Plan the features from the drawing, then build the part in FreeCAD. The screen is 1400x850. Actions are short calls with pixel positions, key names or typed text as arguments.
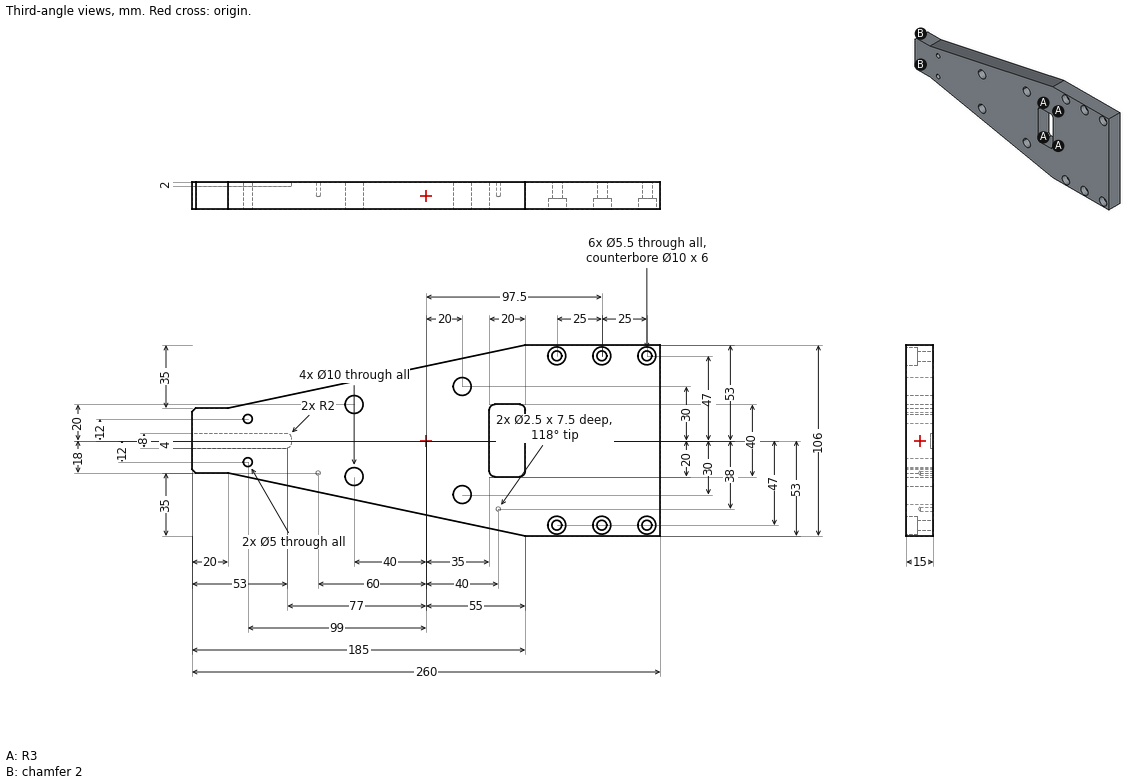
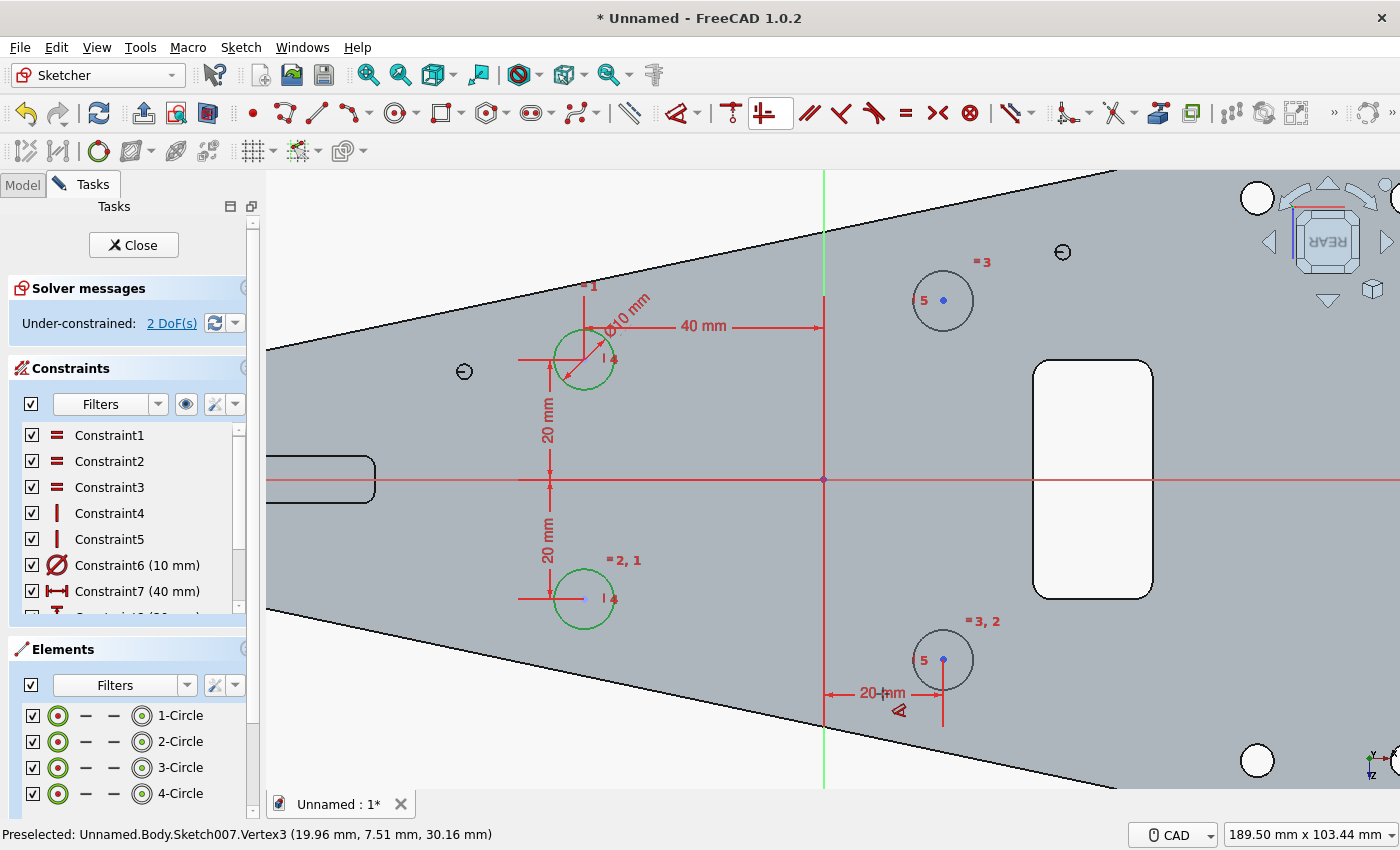
click(943, 660)
click(977, 570)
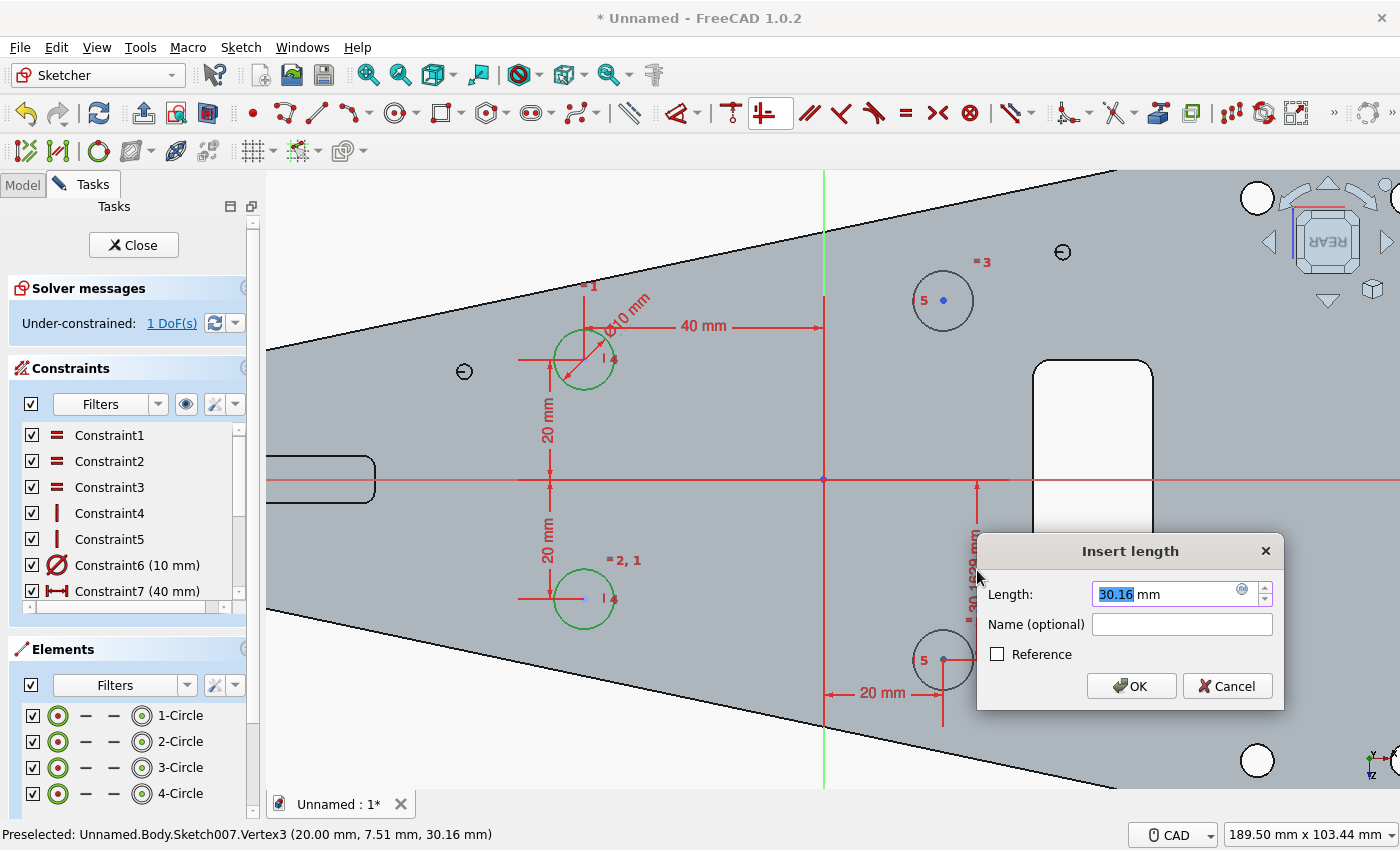
text(30)
key(Return)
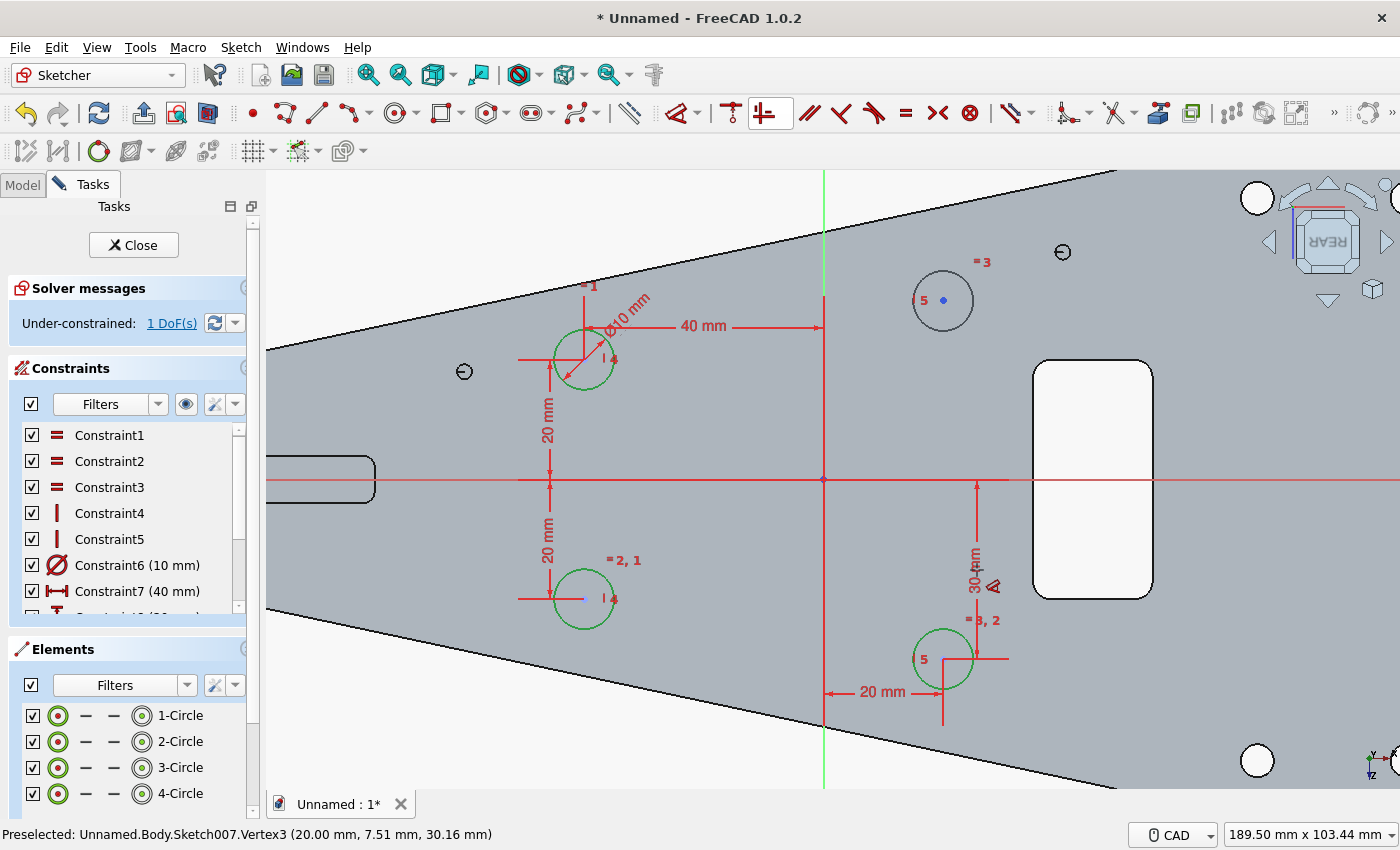
click(943, 301)
click(977, 390)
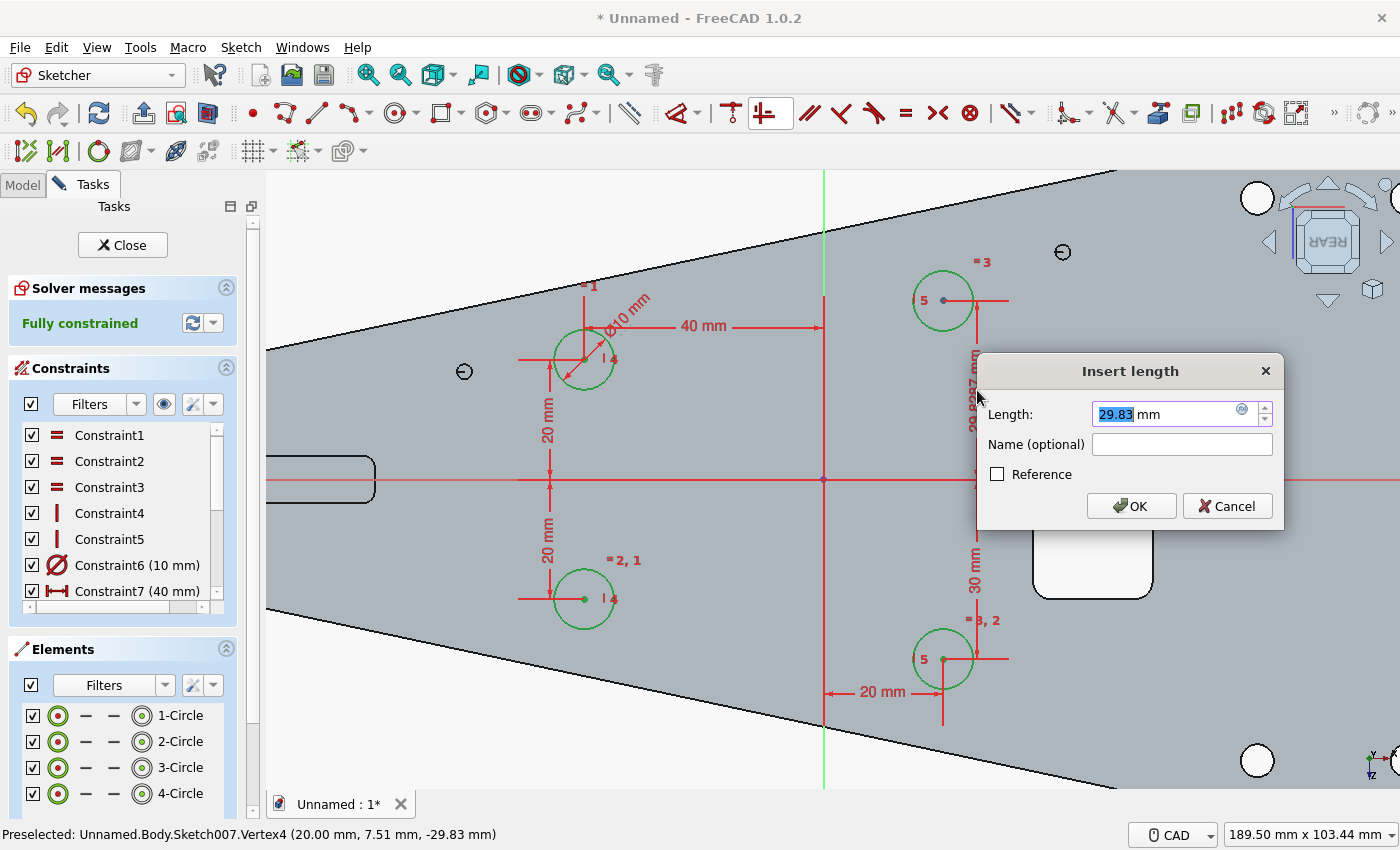
text(30)
key(Return)
key(Escape)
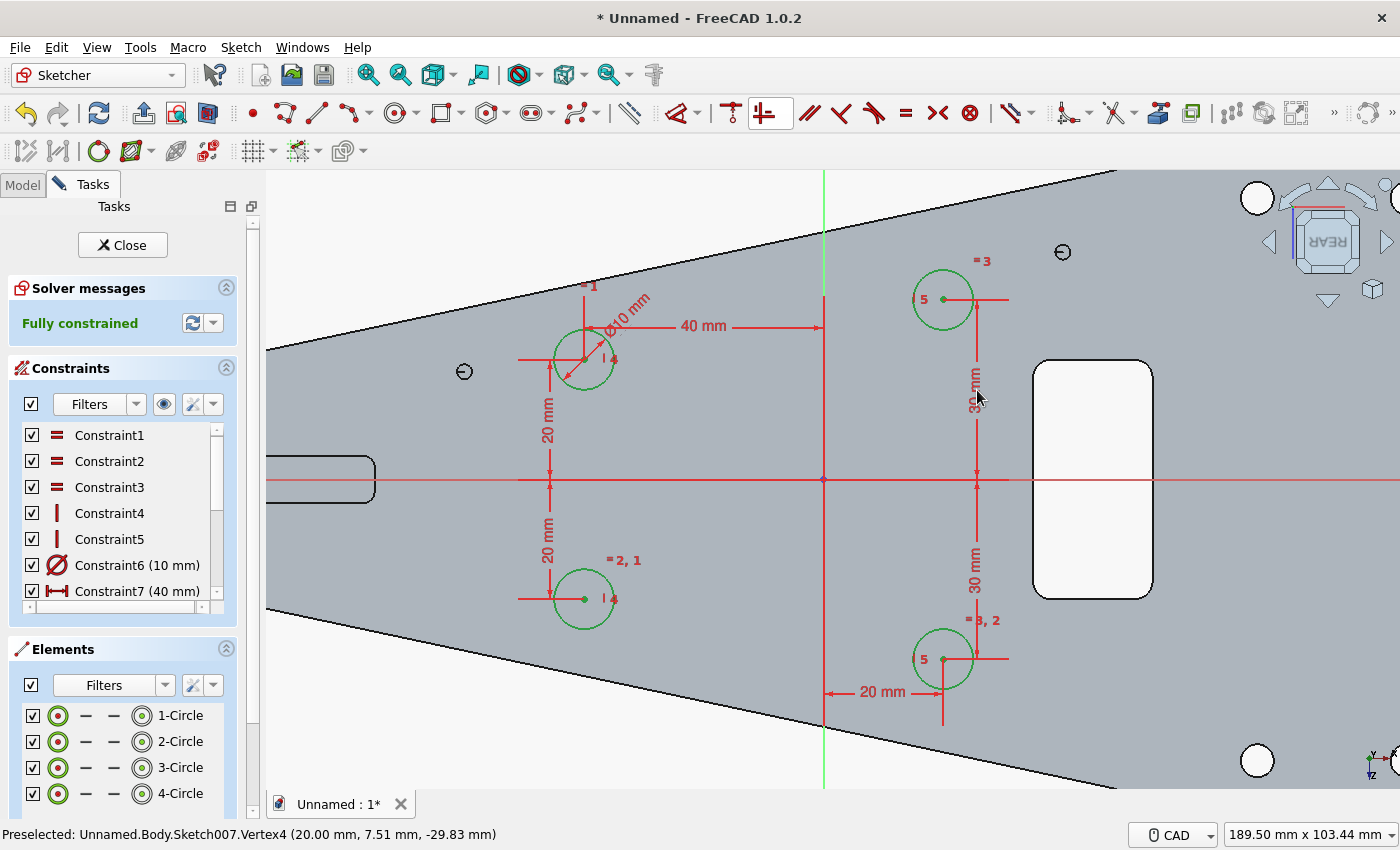
click(123, 245)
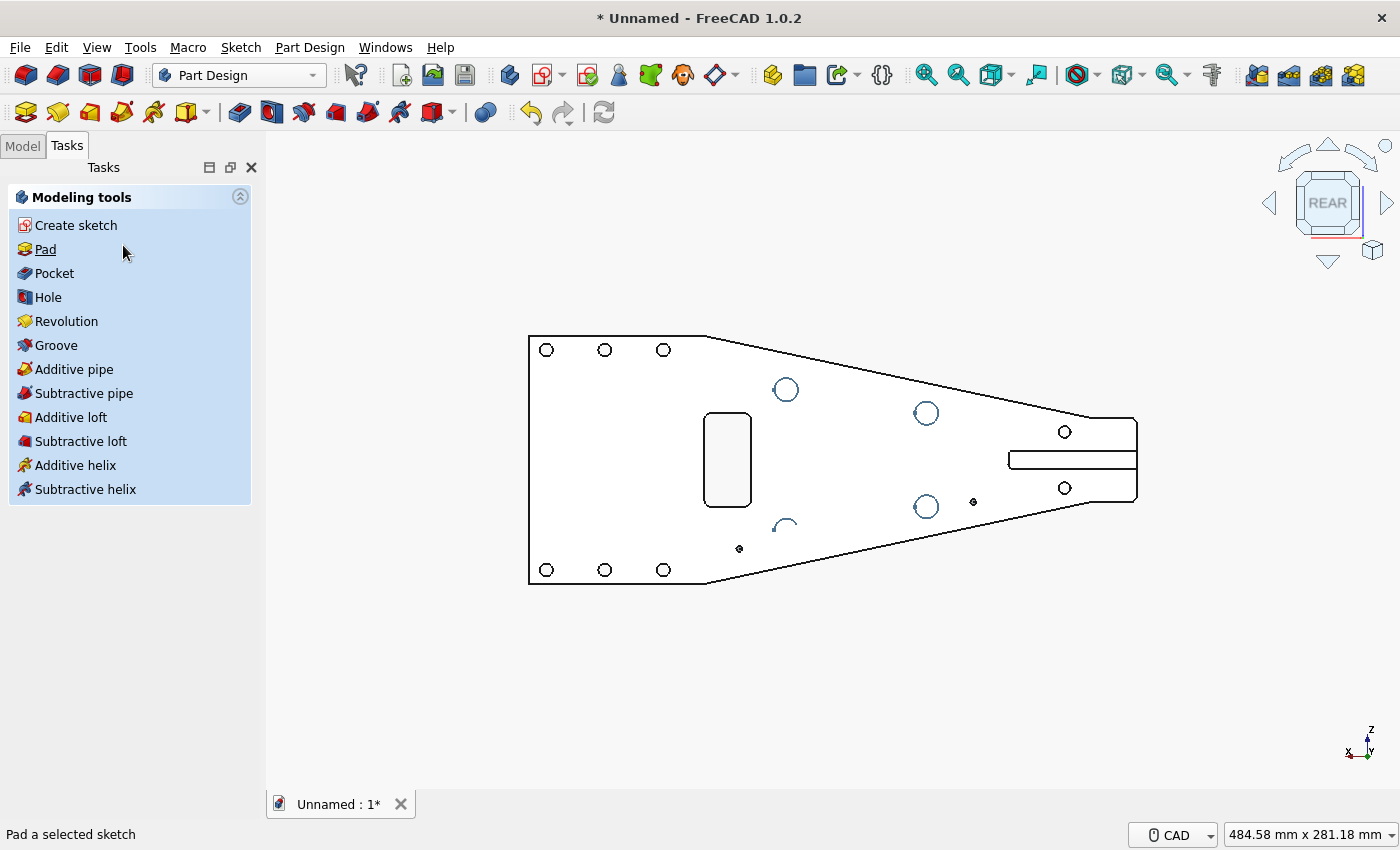
click(272, 112)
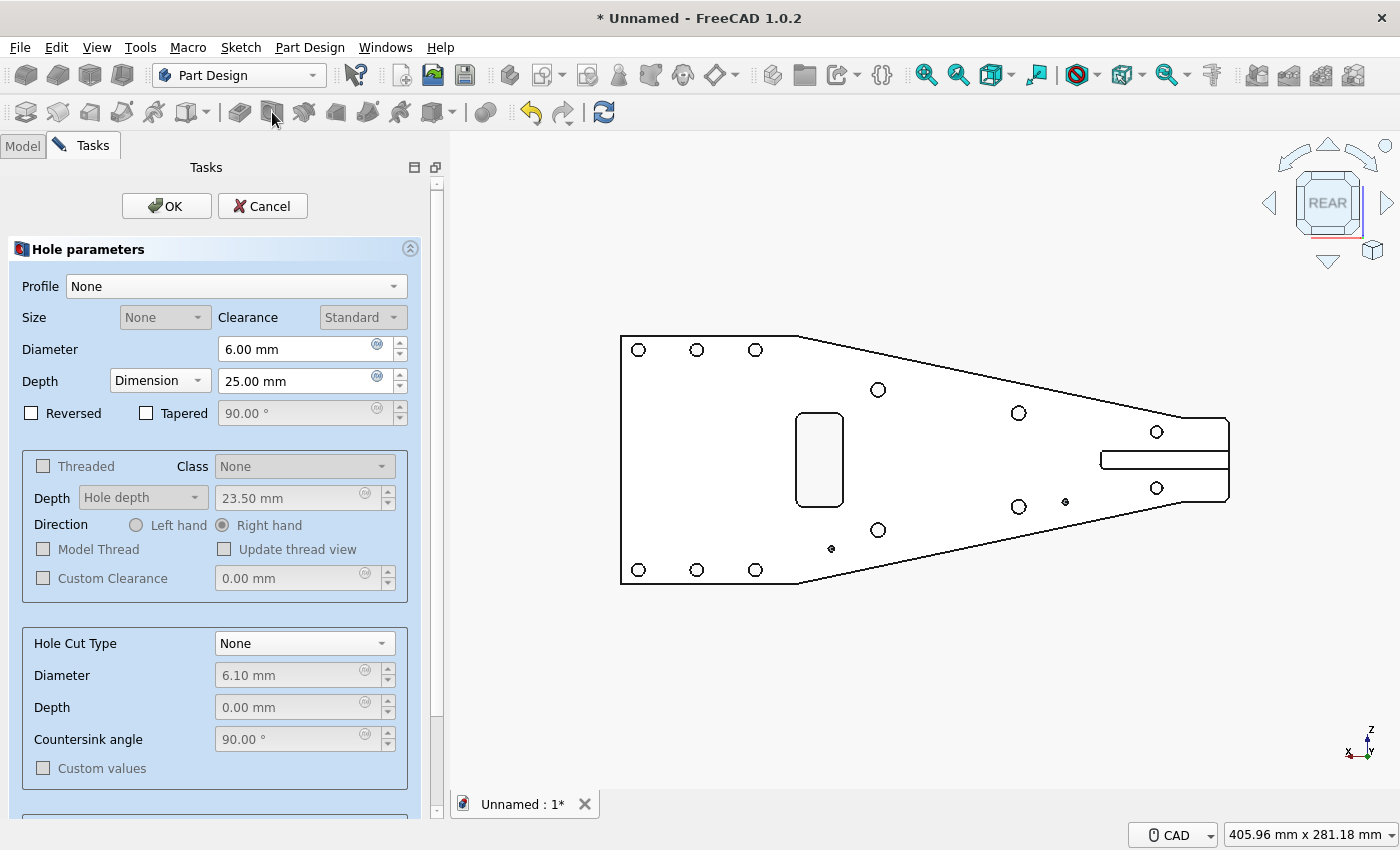
triple_click(305, 349)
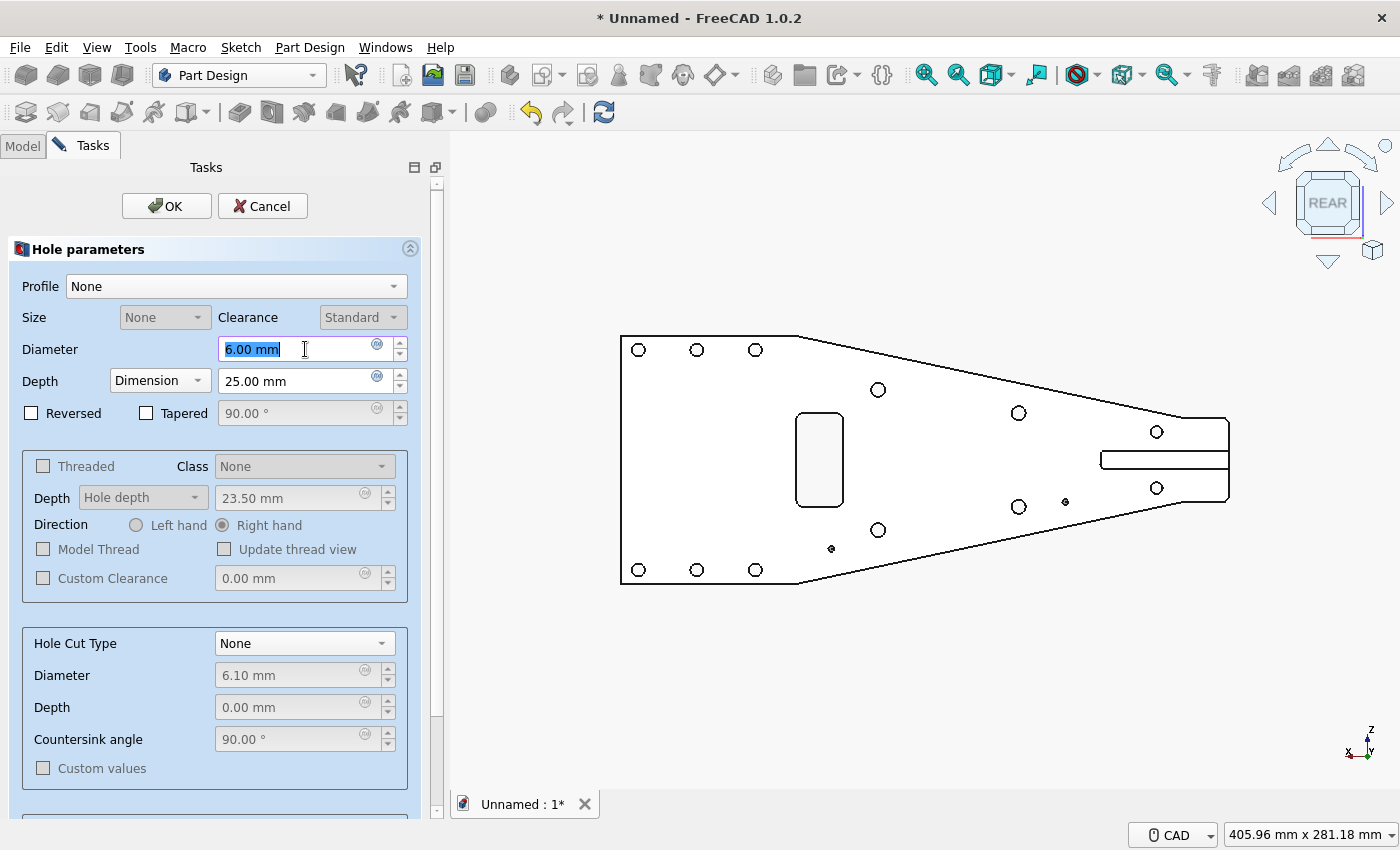
text(10)
key(Tab)